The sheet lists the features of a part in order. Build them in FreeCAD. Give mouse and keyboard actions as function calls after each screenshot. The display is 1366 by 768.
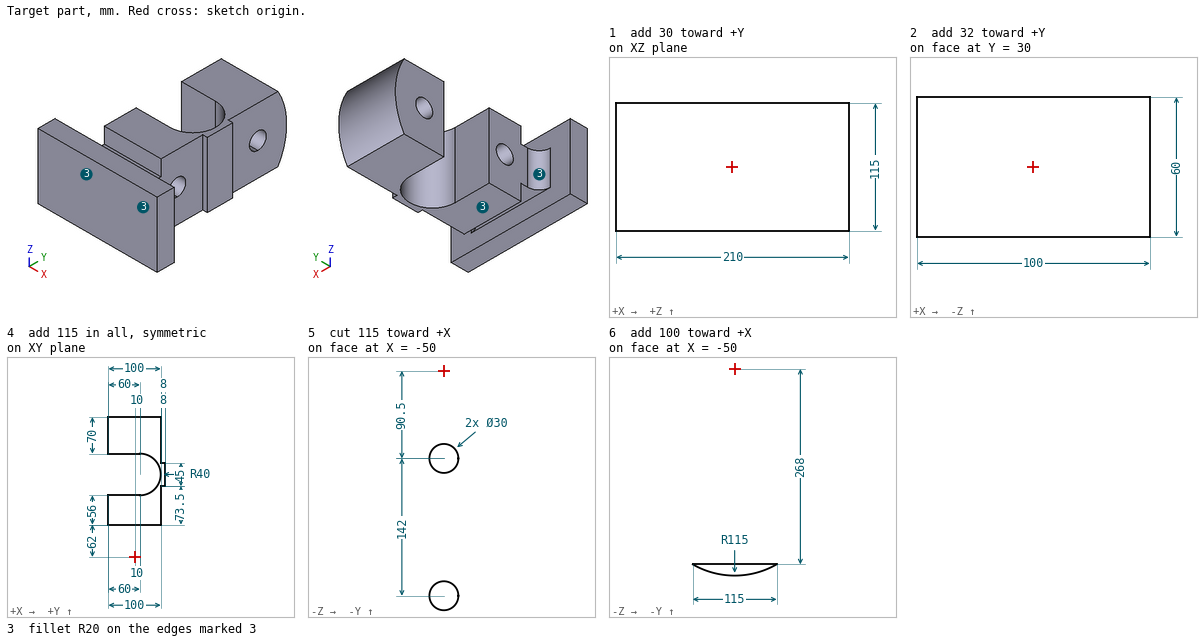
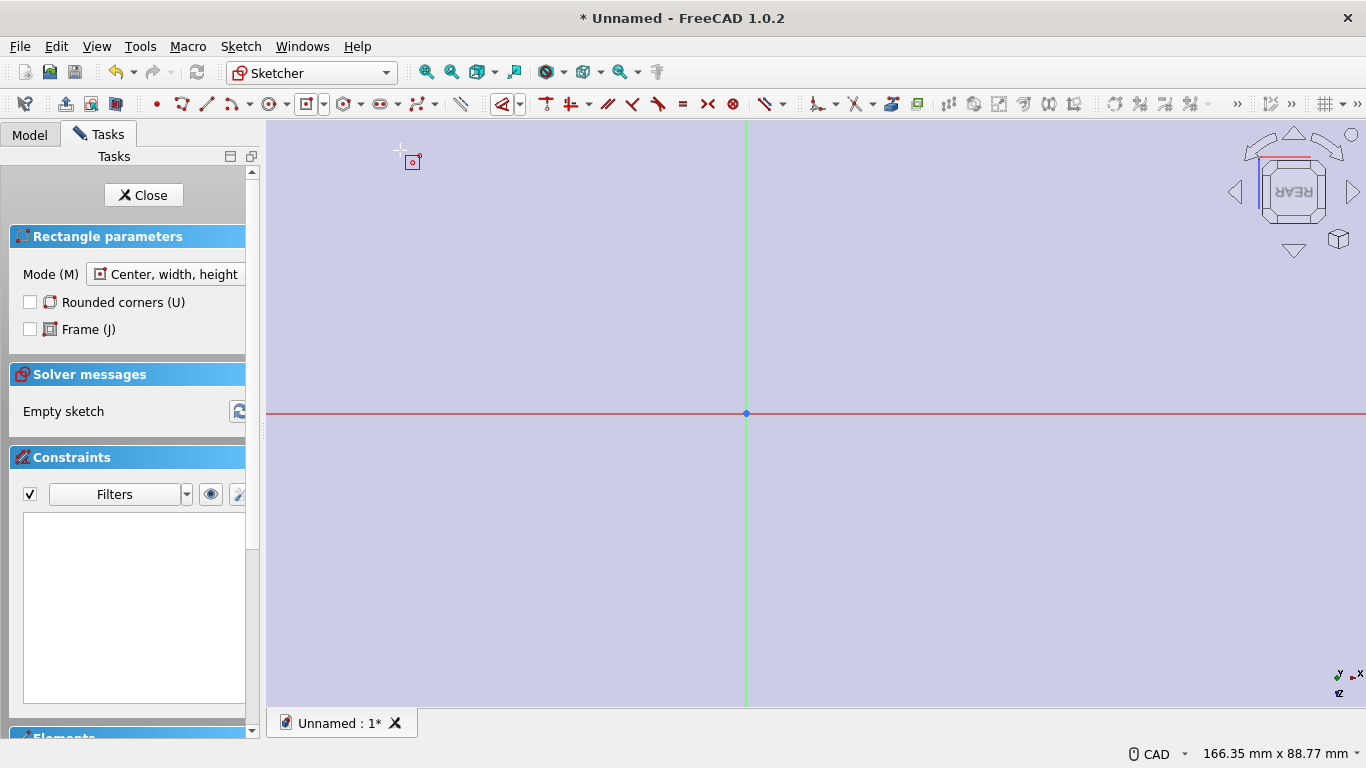
click(746, 413)
move(1077, 215)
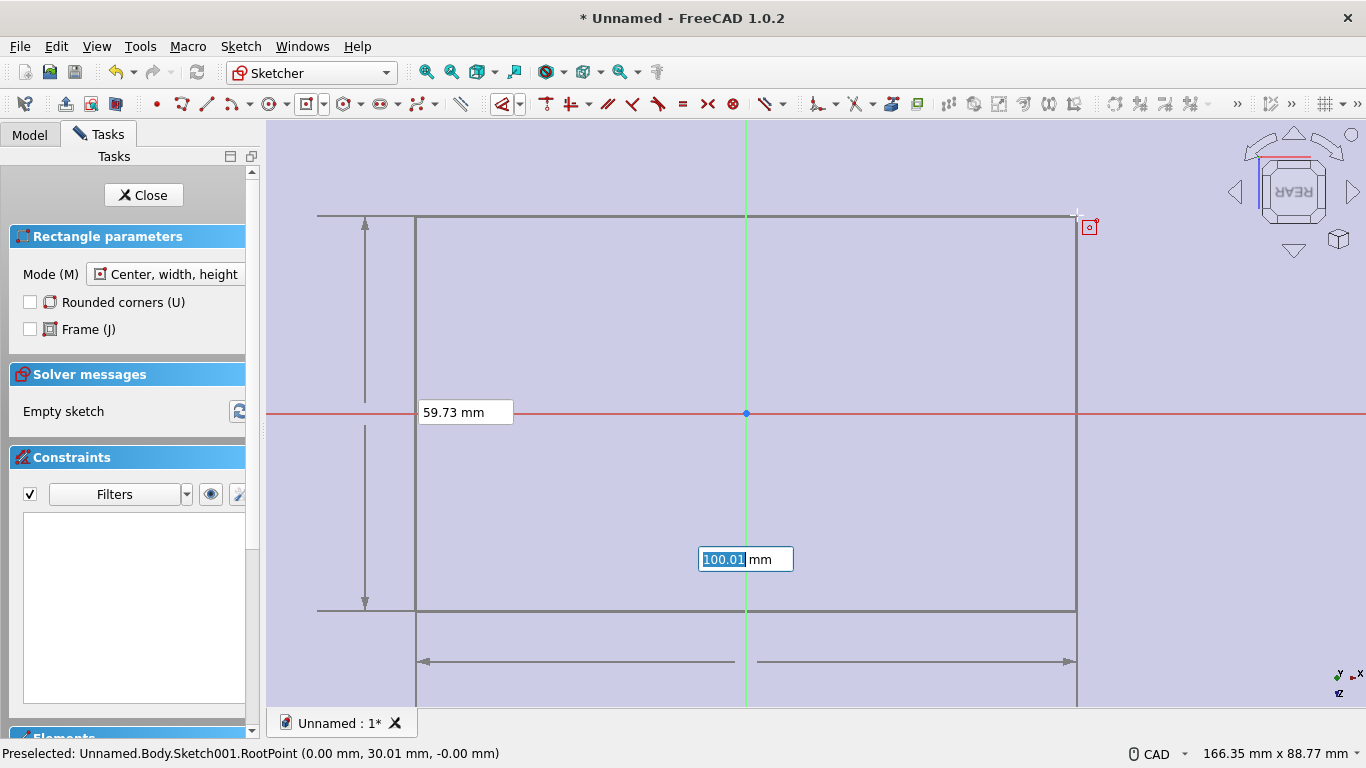
text(100)
key(Tab)
text(60)
key(Return)
key(Escape)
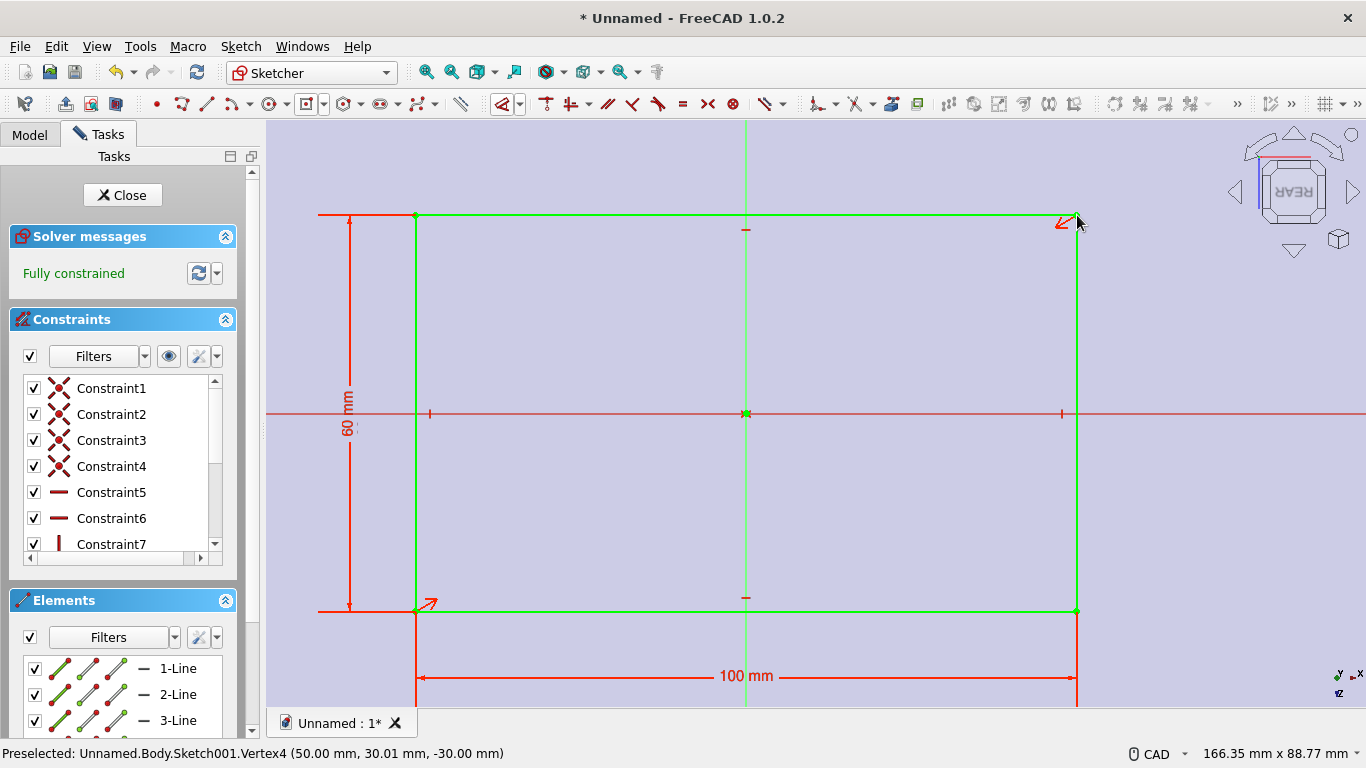
click(123, 195)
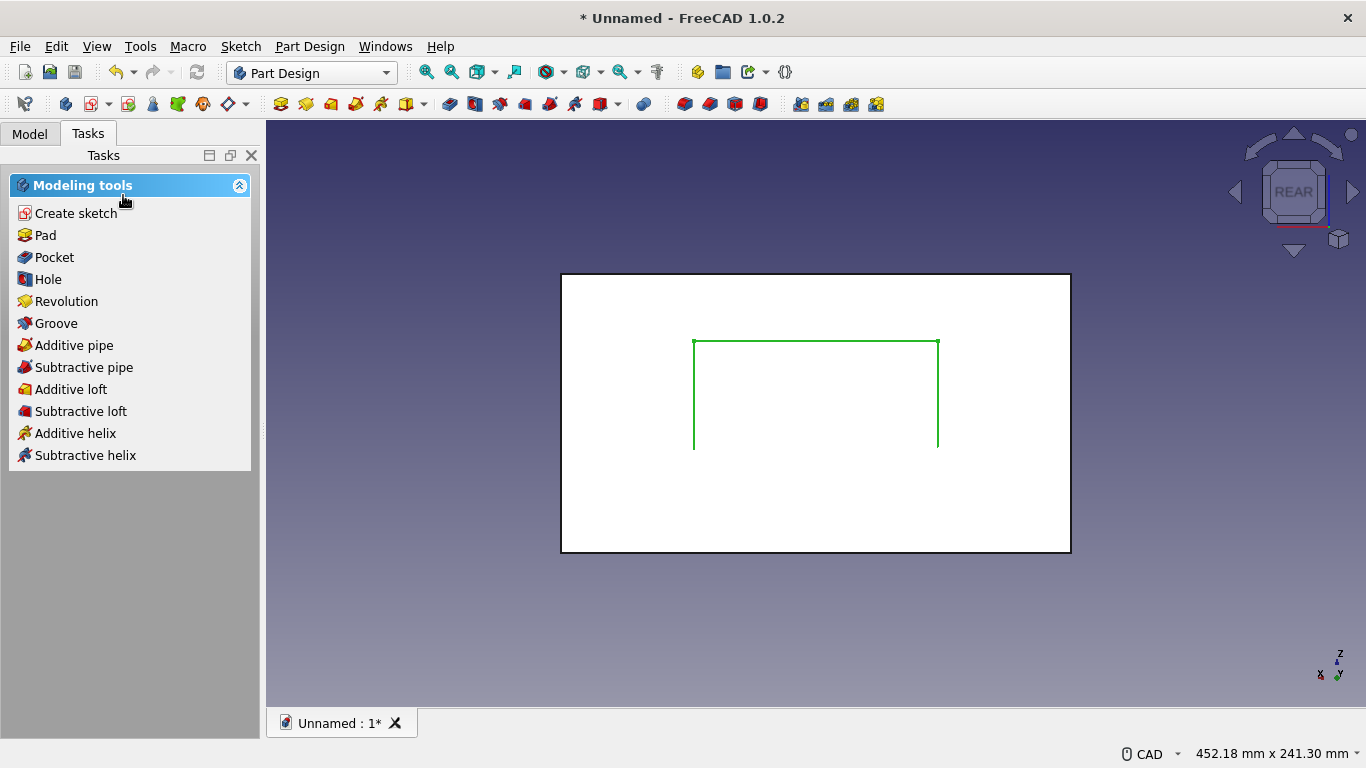
click(281, 104)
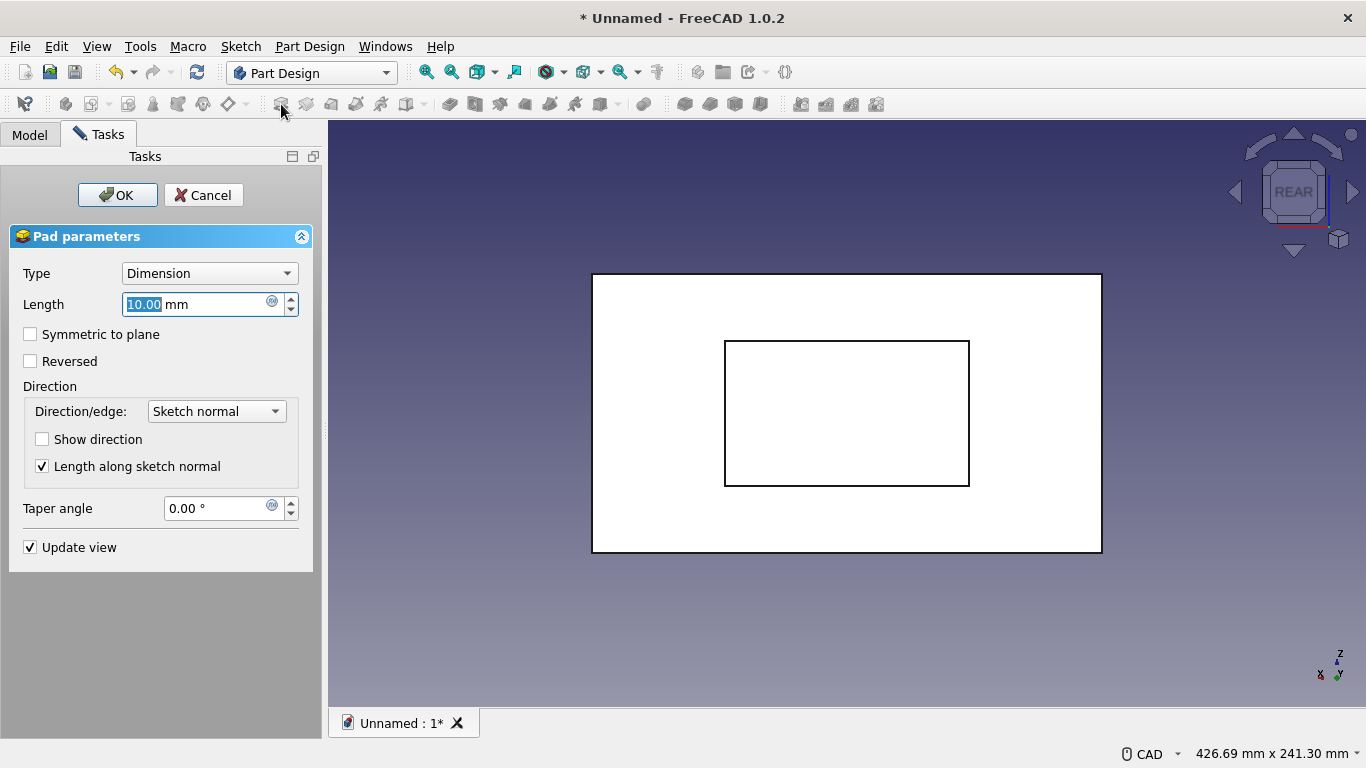
text(32)
key(Tab)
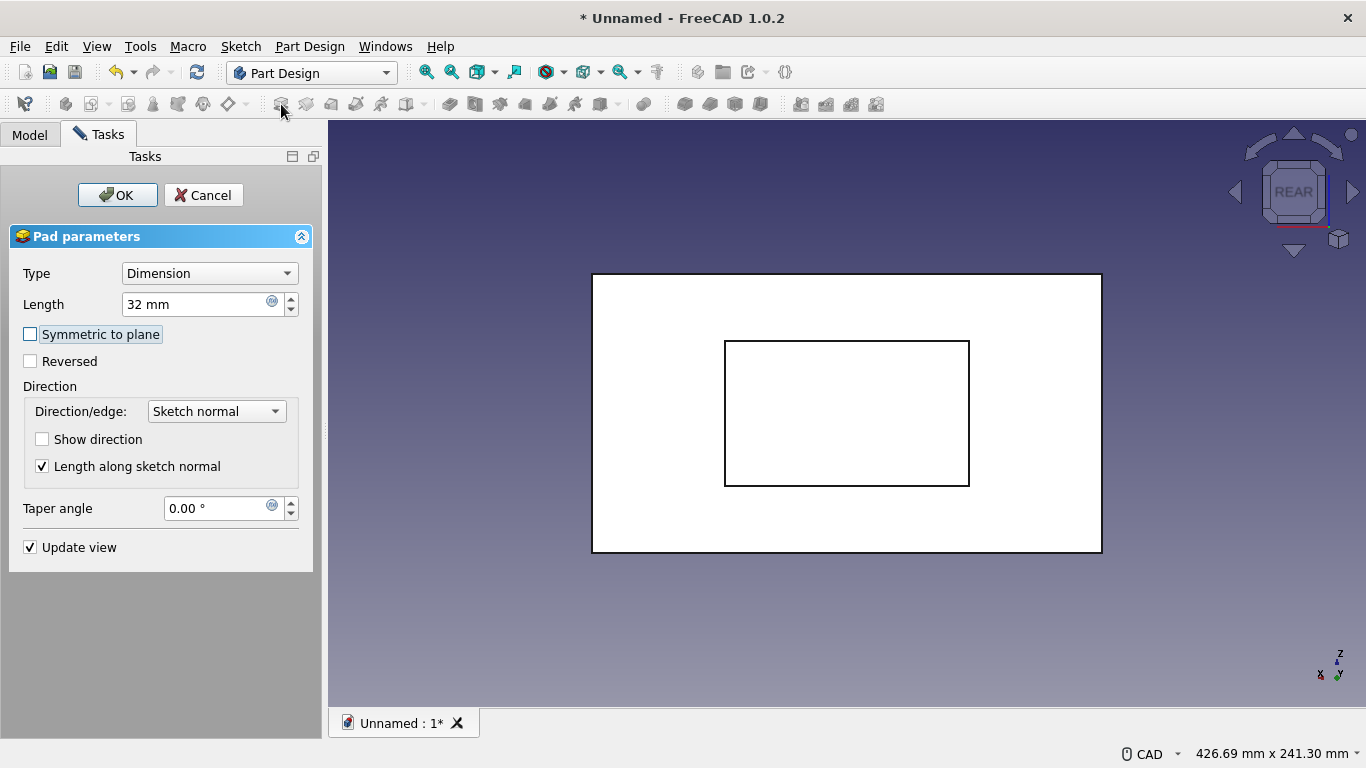
click(118, 195)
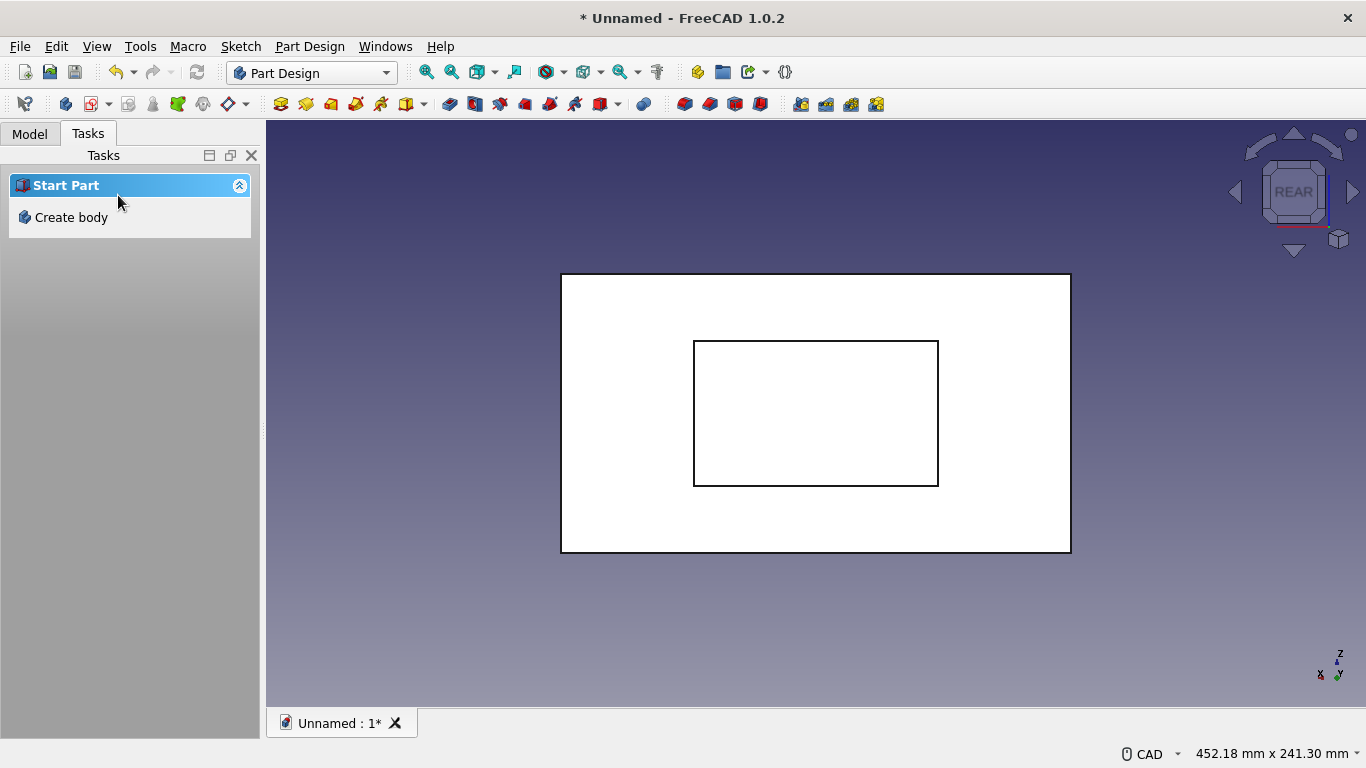
key(0)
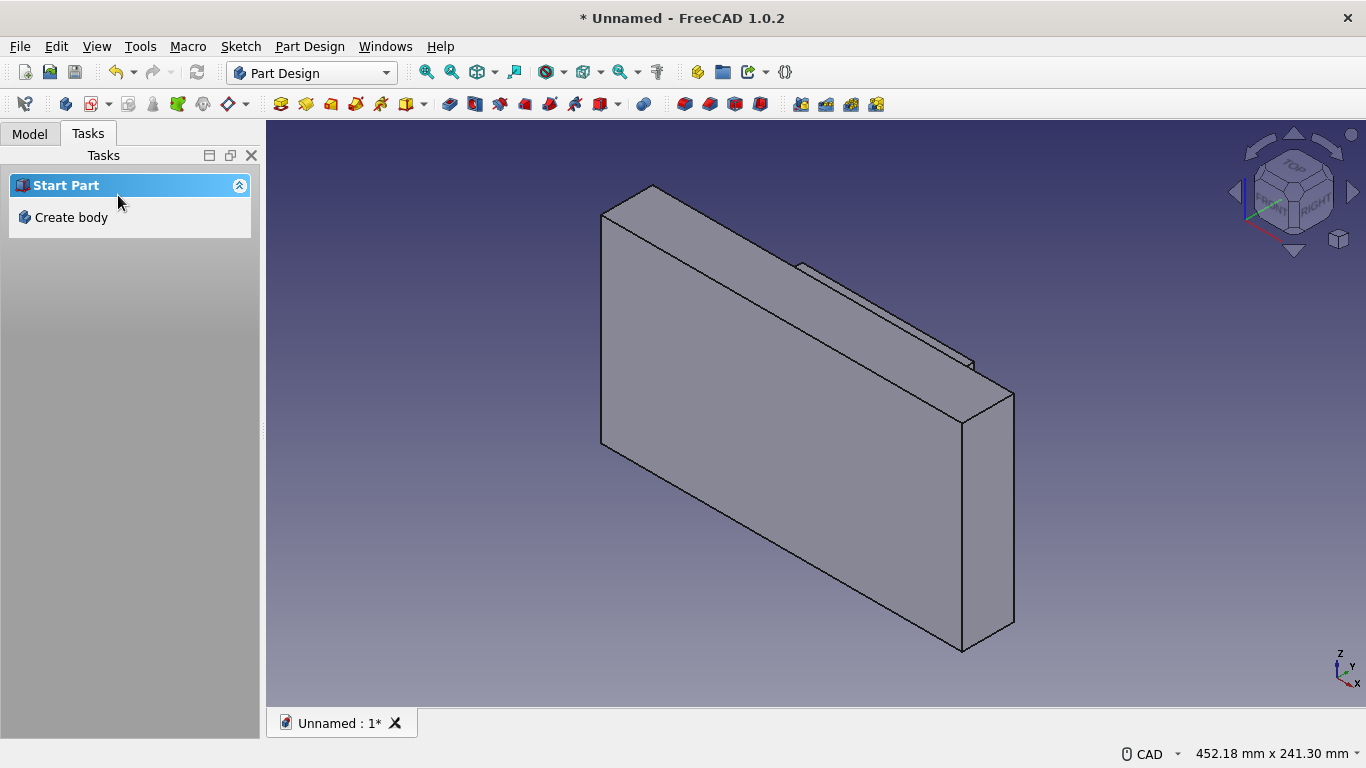
key(2)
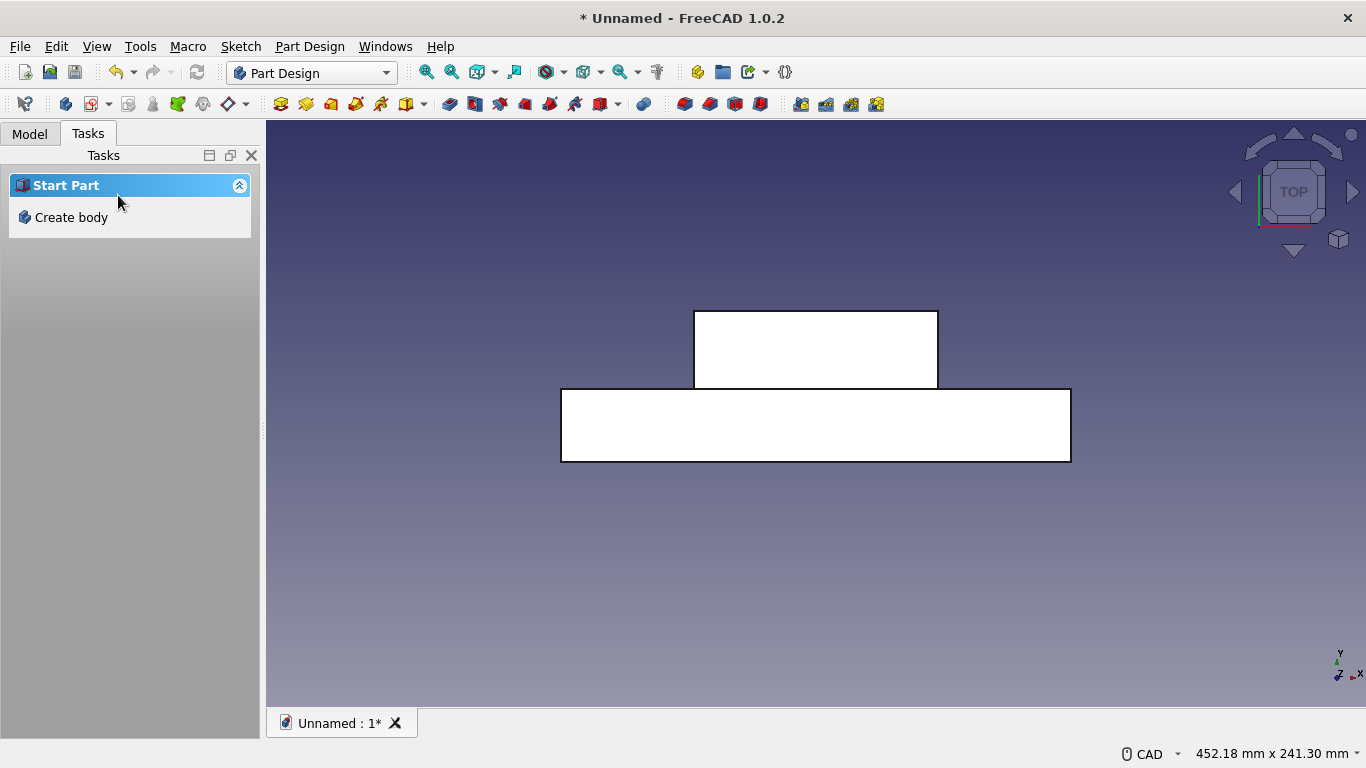
key(1)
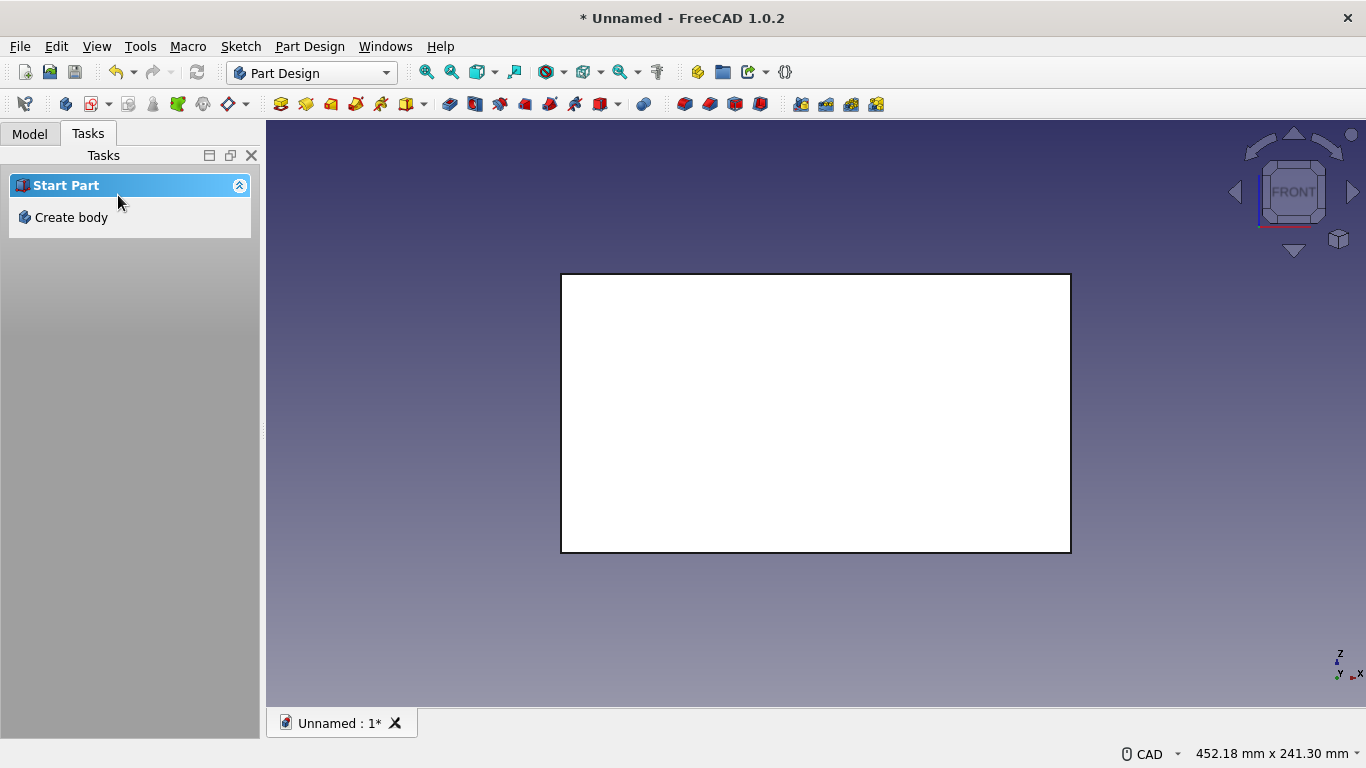
key(3)